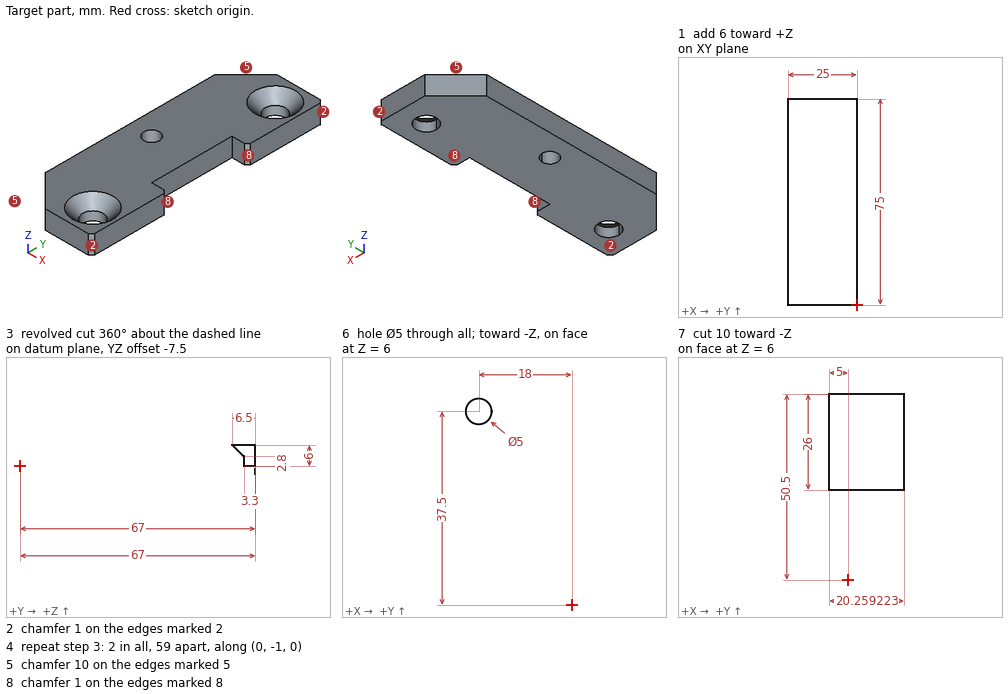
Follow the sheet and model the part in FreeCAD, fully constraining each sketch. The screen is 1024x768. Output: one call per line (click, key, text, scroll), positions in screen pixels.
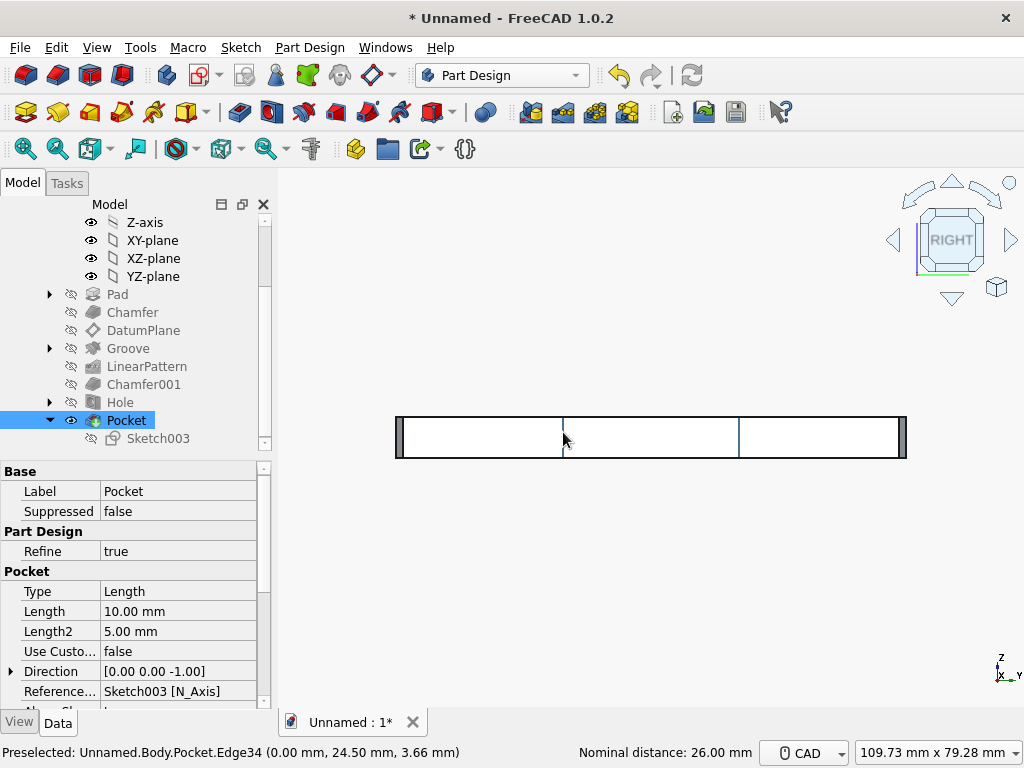
click(58, 76)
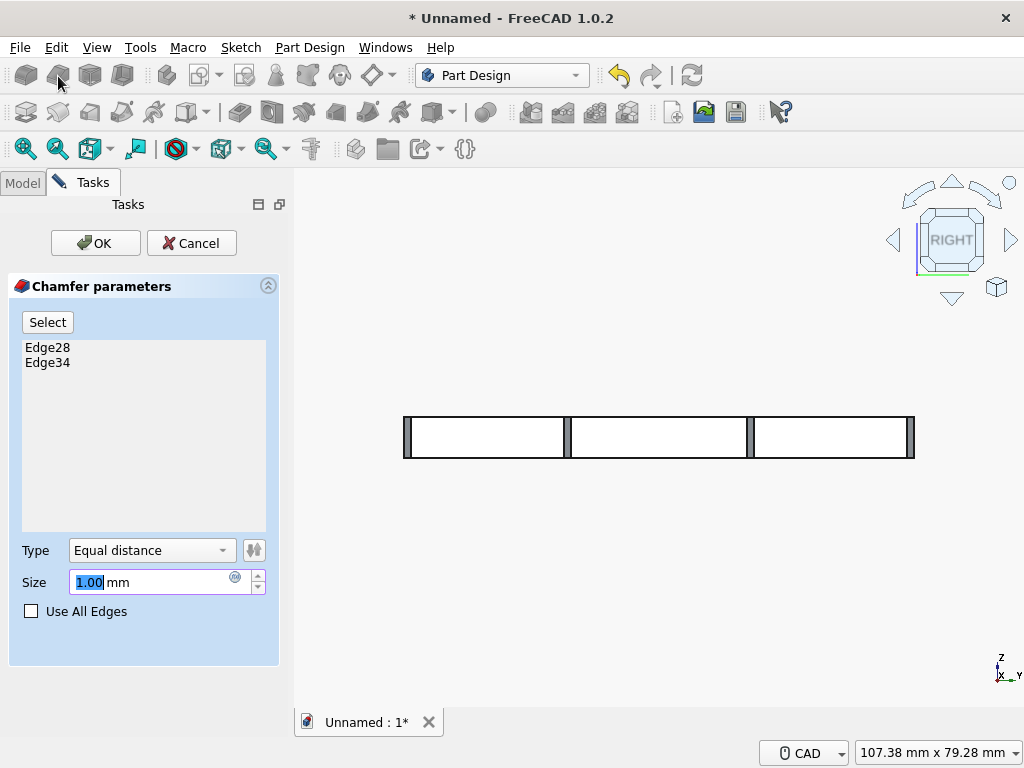
text(1)
key(Tab)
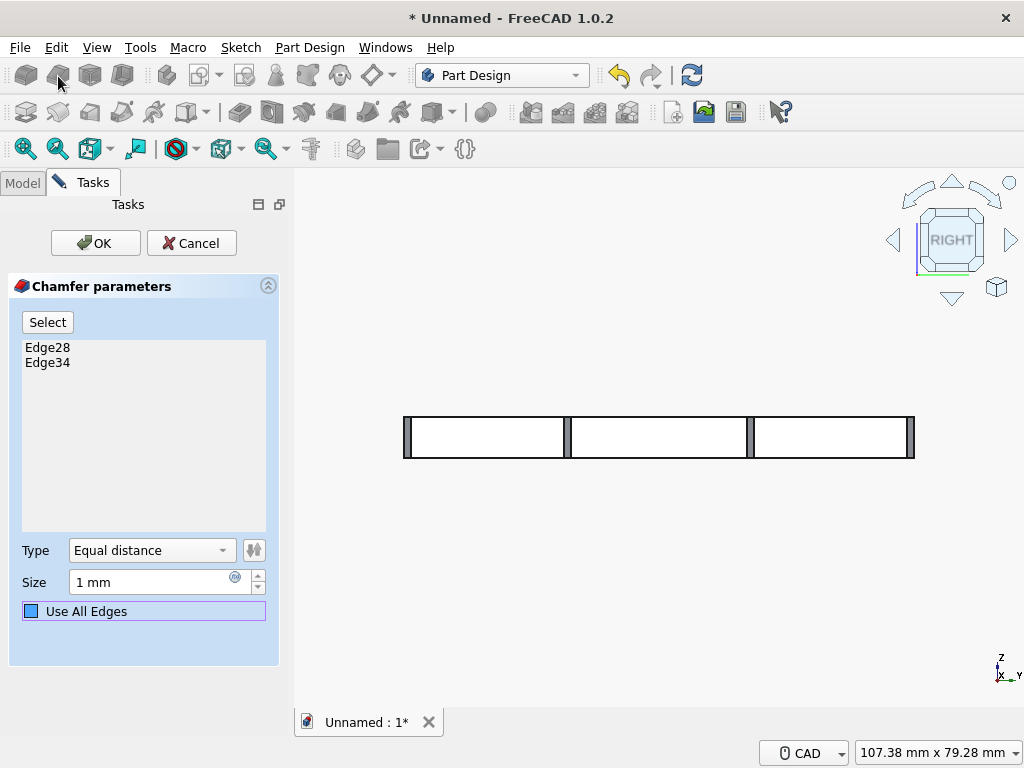
click(96, 243)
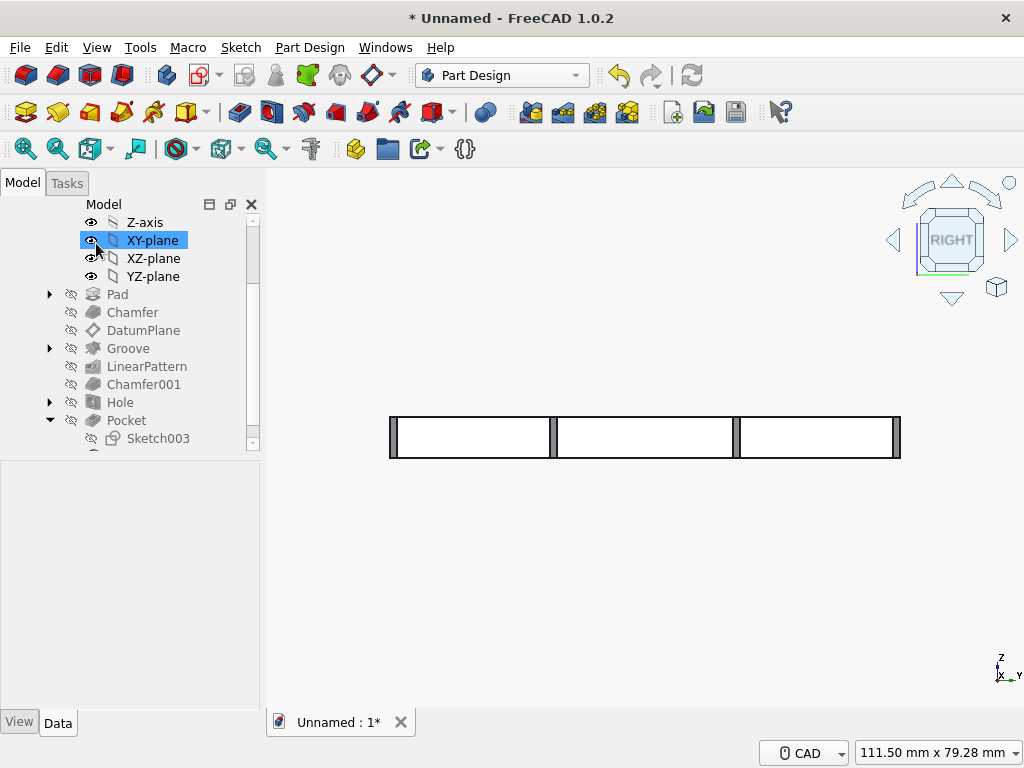
key(0)